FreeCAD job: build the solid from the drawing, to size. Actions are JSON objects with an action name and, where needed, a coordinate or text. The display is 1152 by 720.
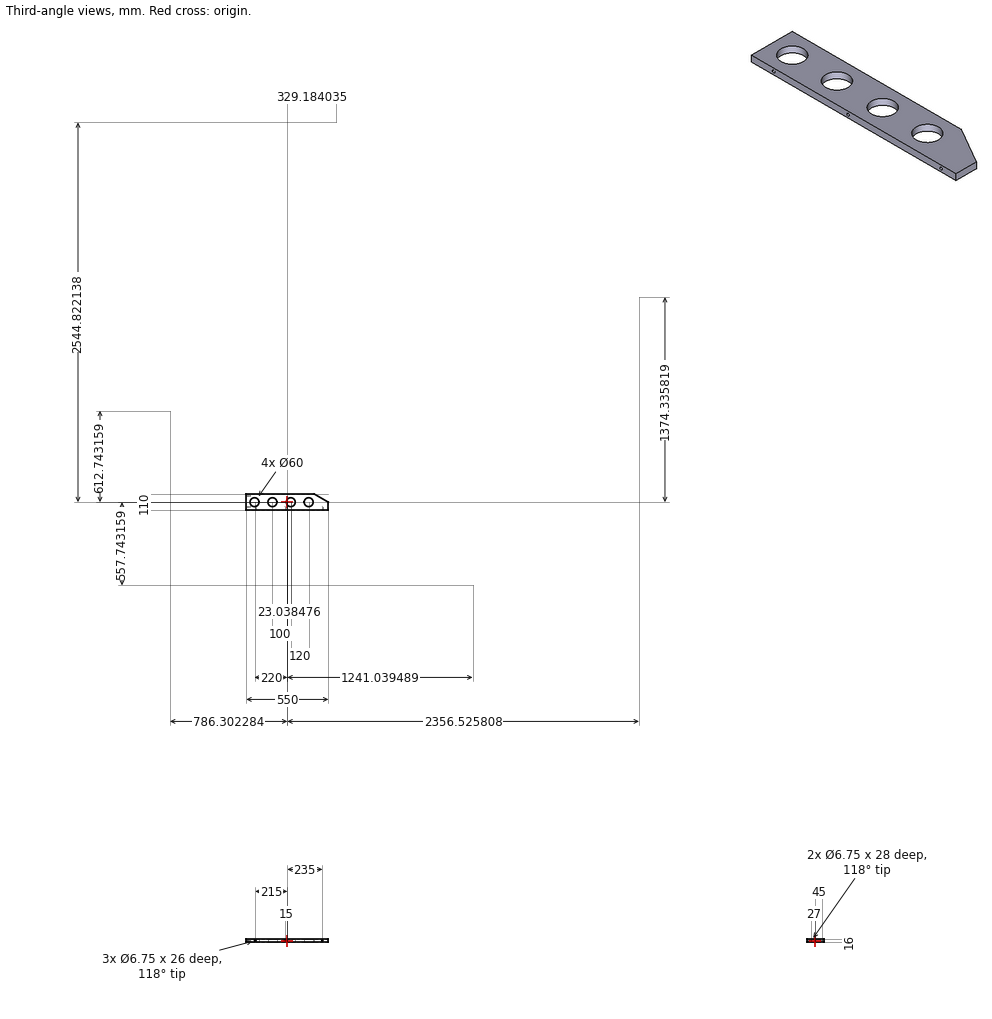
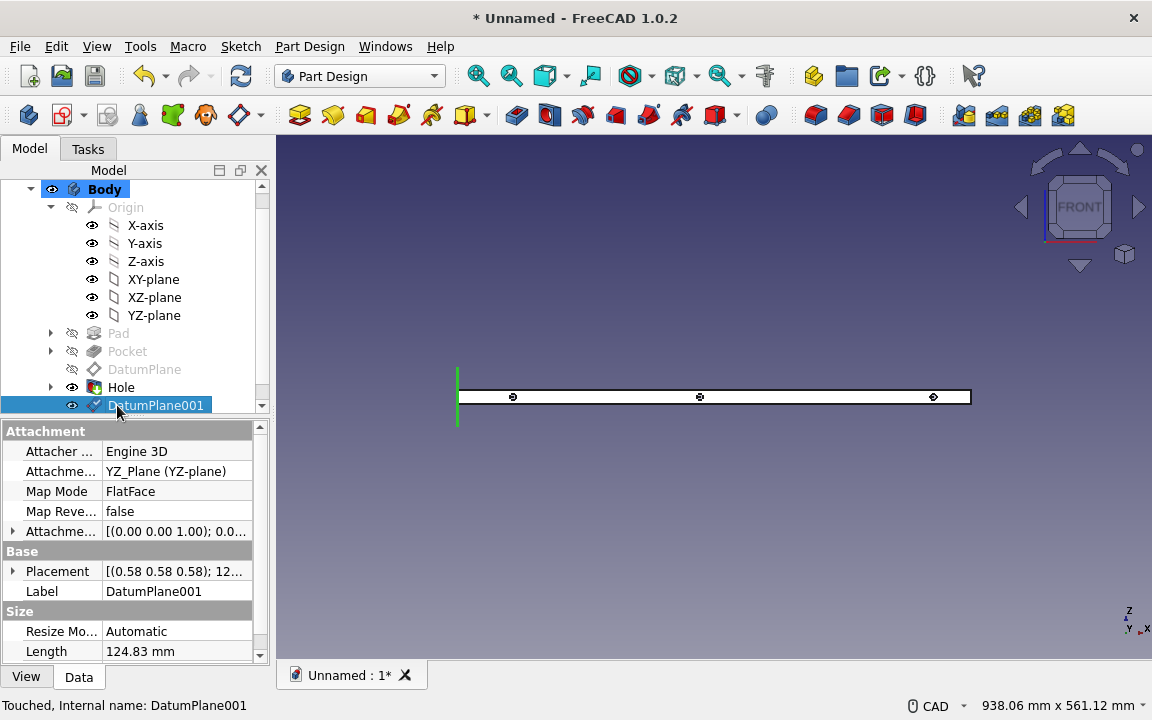
{"action": "left_click", "coordinate": [62, 116]}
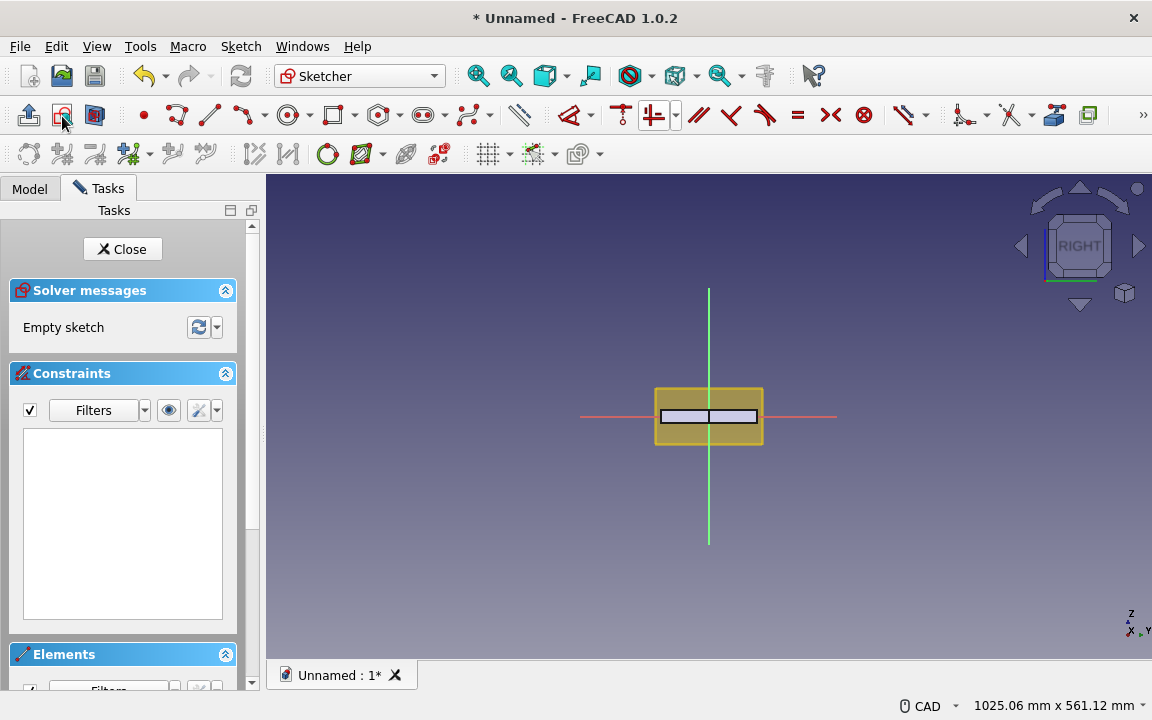
{"action": "key", "text": "q s"}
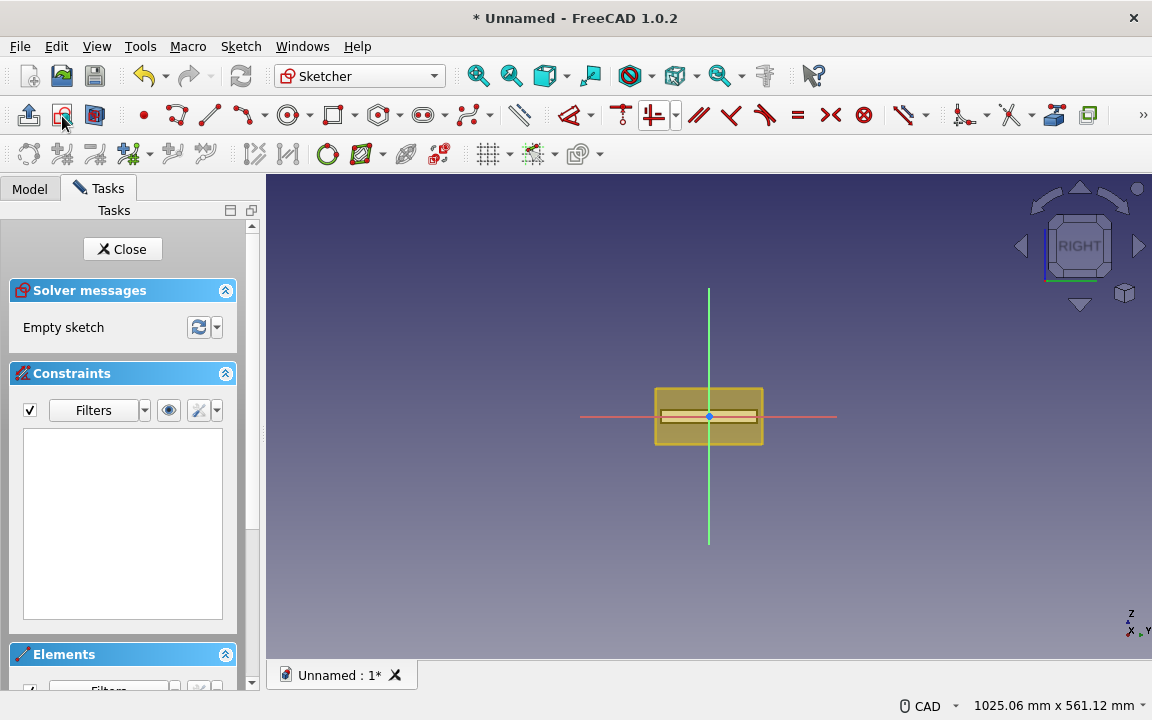
{"action": "scroll", "coordinate": [729, 416], "scroll_direction": "up", "scroll_amount": 10}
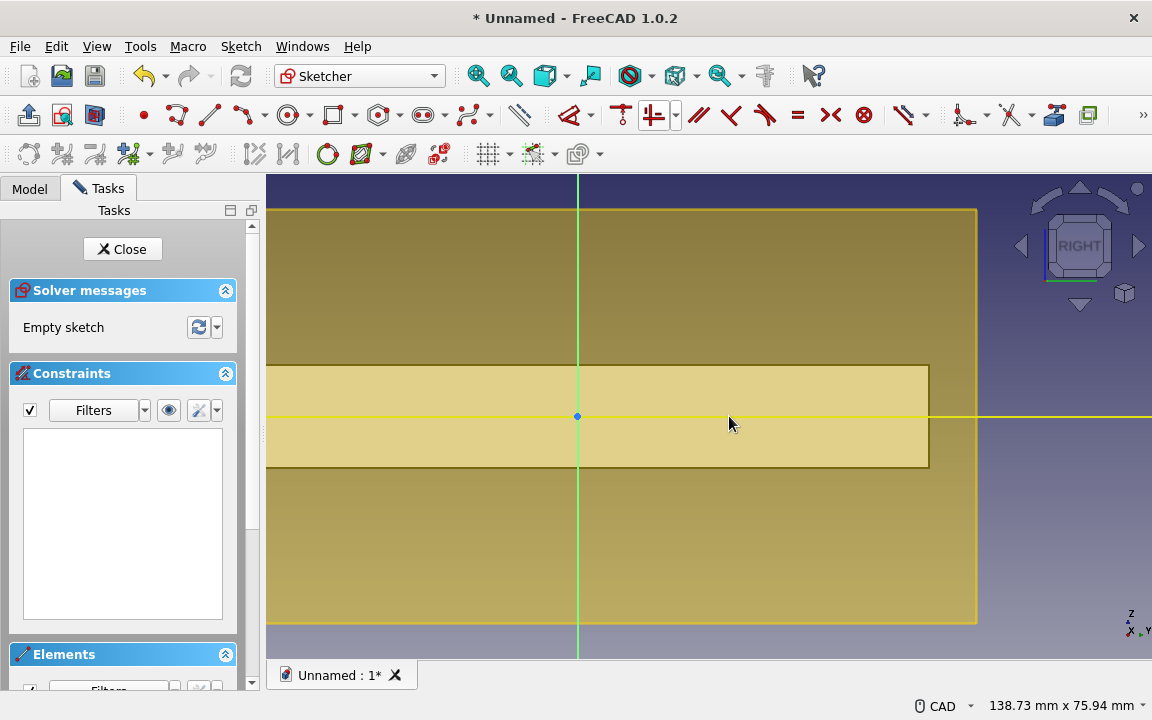
{"action": "key", "text": "g c"}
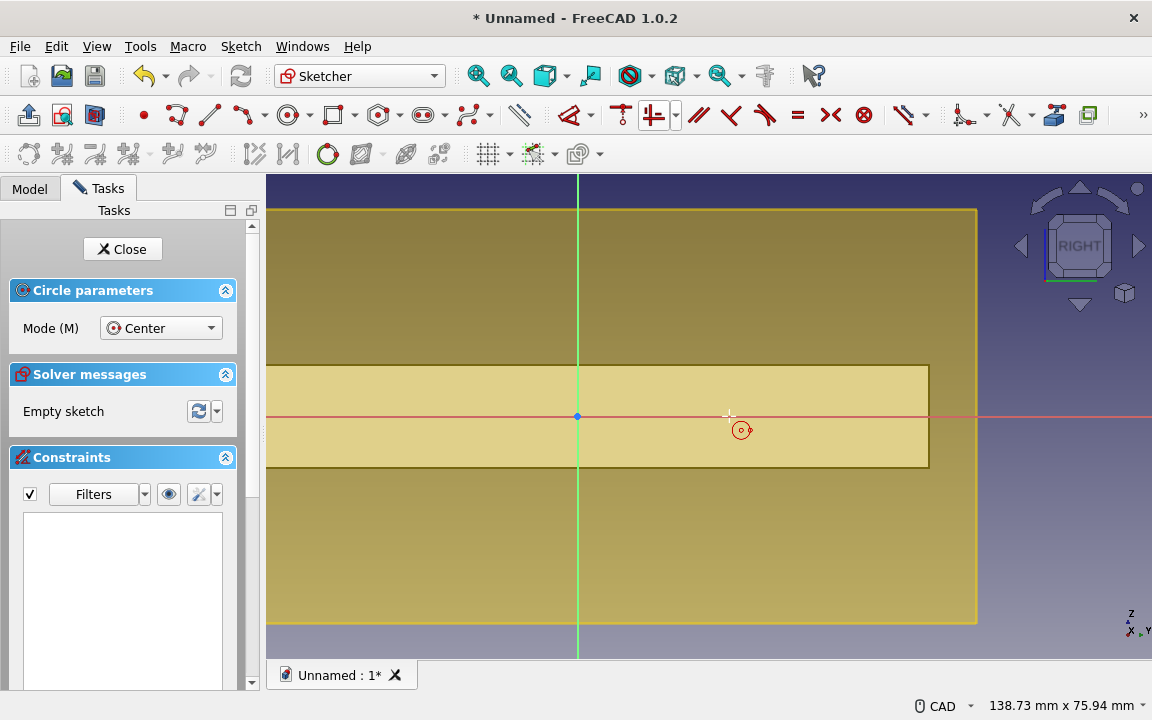
{"action": "left_click", "coordinate": [405, 416]}
{"action": "mouse_move", "coordinate": [421, 401]}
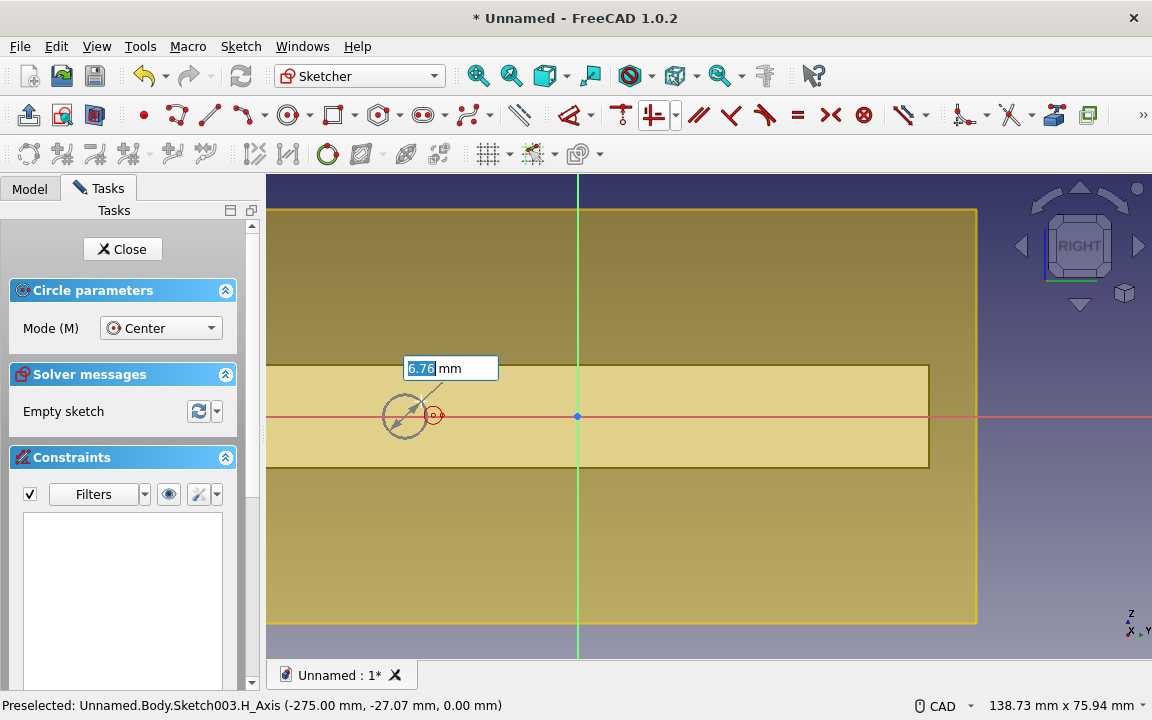
{"action": "type", "text": "6.75"}
{"action": "key", "text": "Return"}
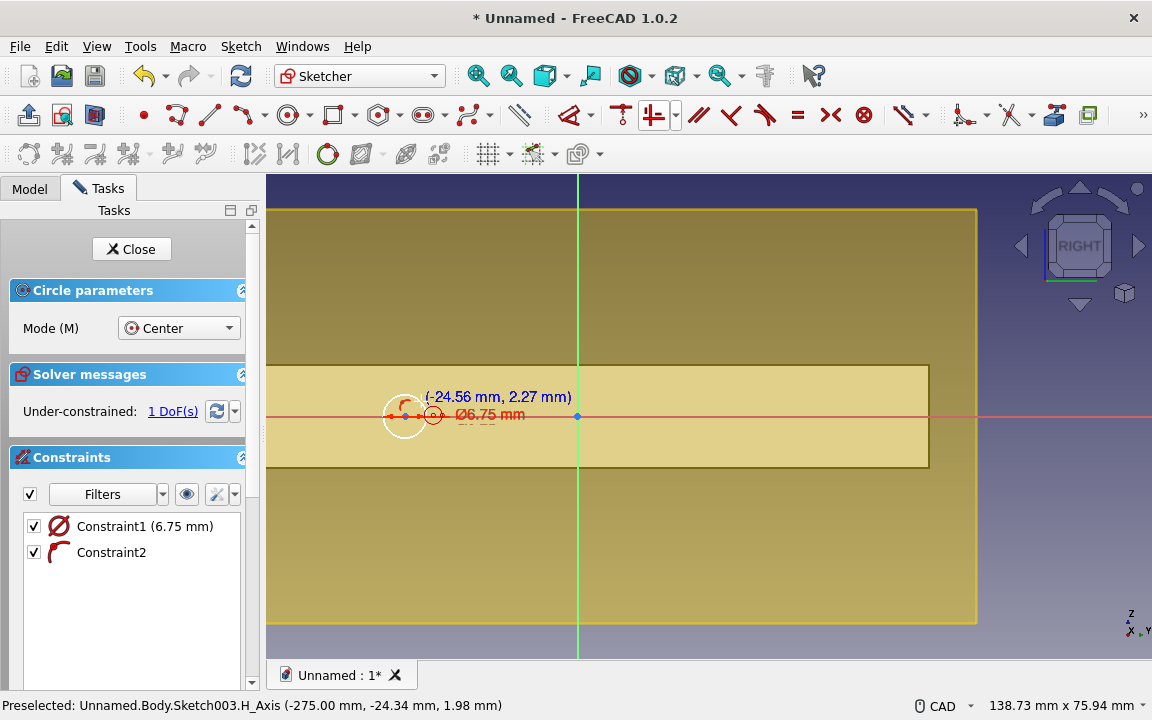
{"action": "left_click", "coordinate": [865, 416]}
{"action": "mouse_move", "coordinate": [881, 401]}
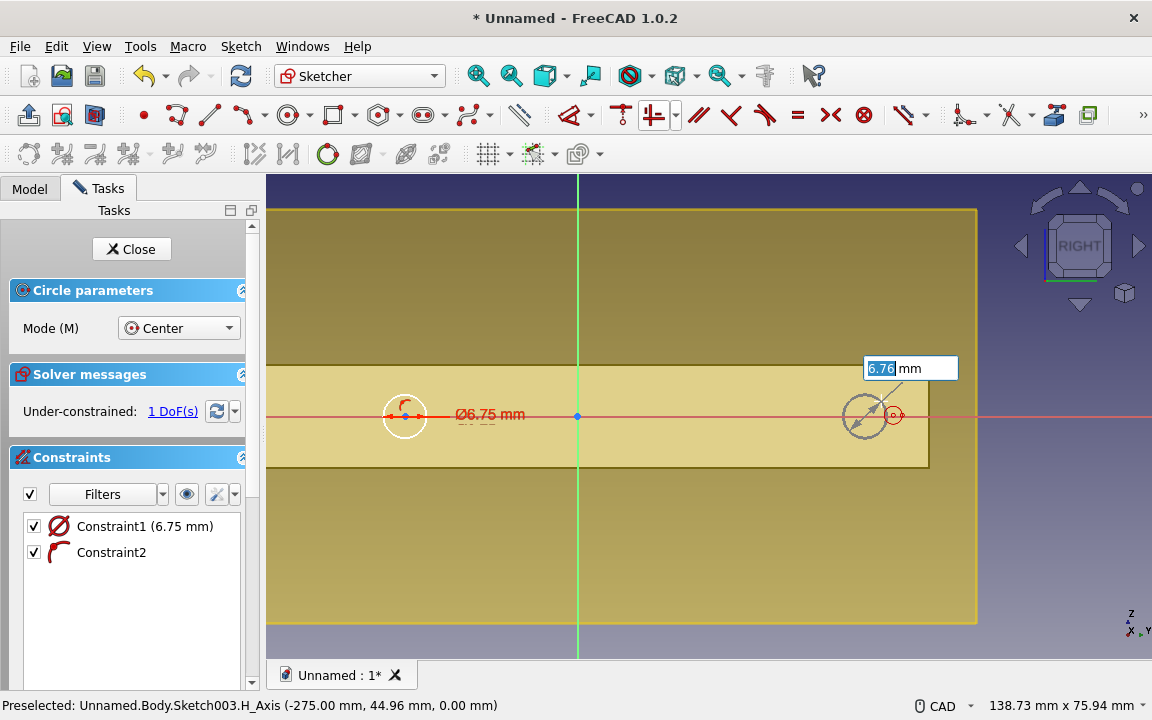
{"action": "type", "text": "6.75"}
{"action": "key", "text": "Return"}
{"action": "key", "text": "Escape"}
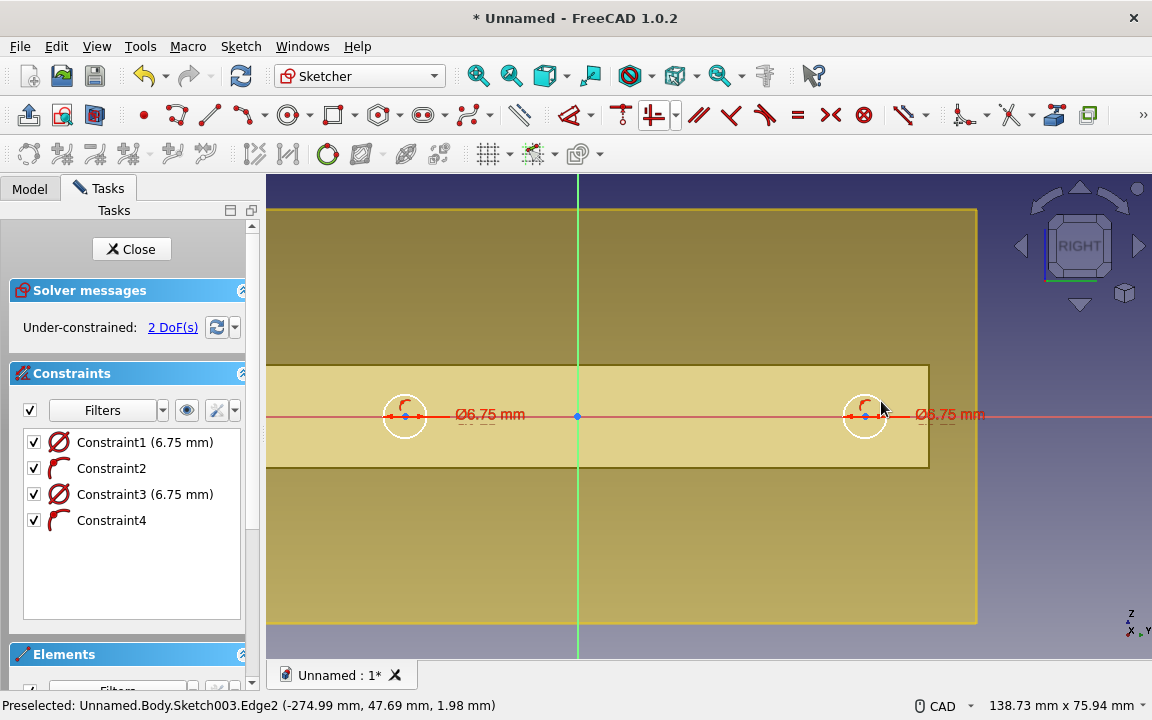
{"action": "key", "text": "d"}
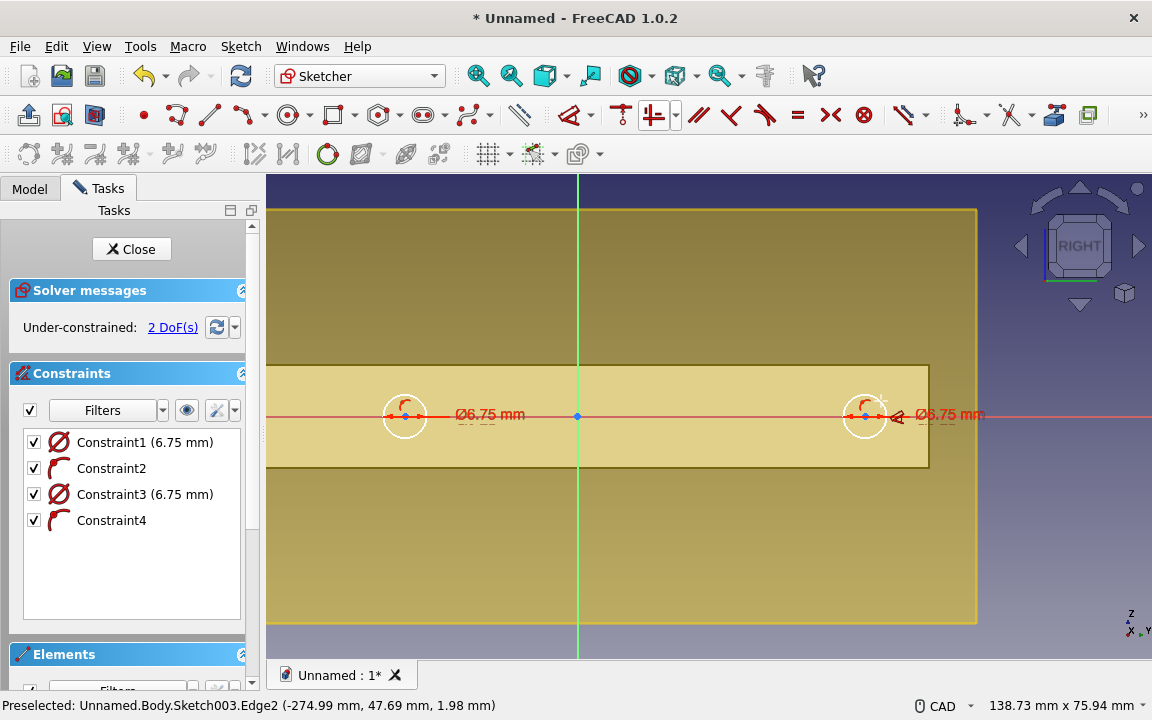
{"action": "left_click", "coordinate": [405, 416]}
{"action": "left_click", "coordinate": [491, 450]}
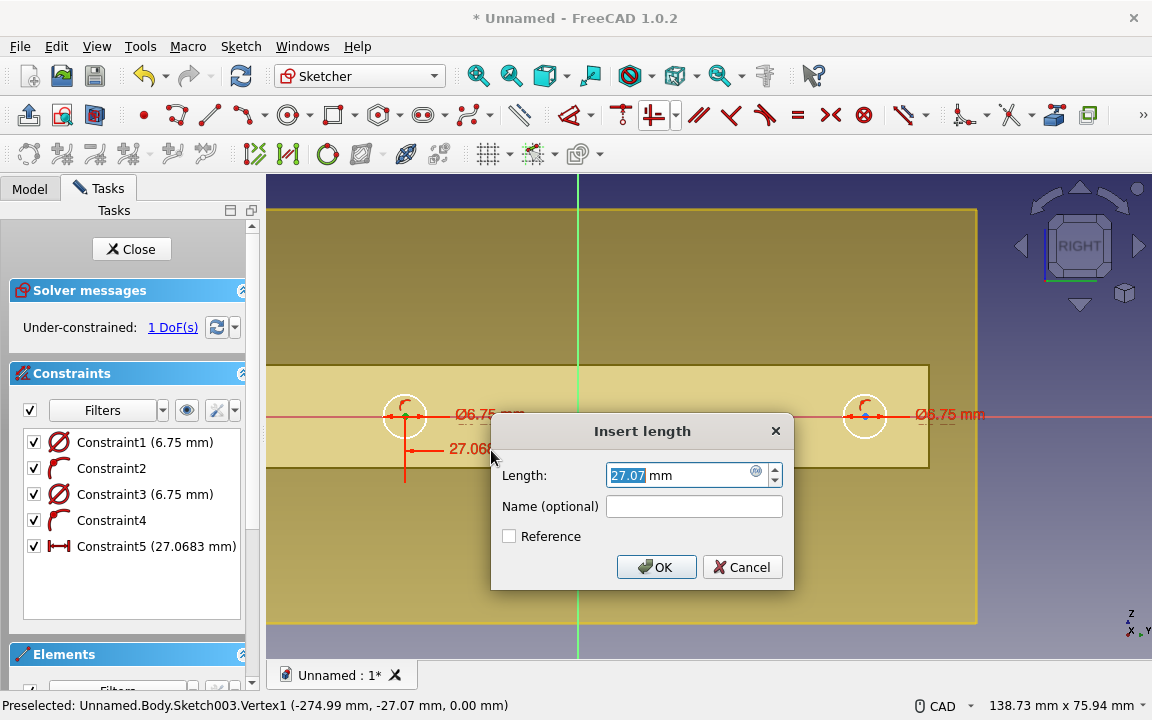
{"action": "type", "text": "27"}
{"action": "key", "text": "Return"}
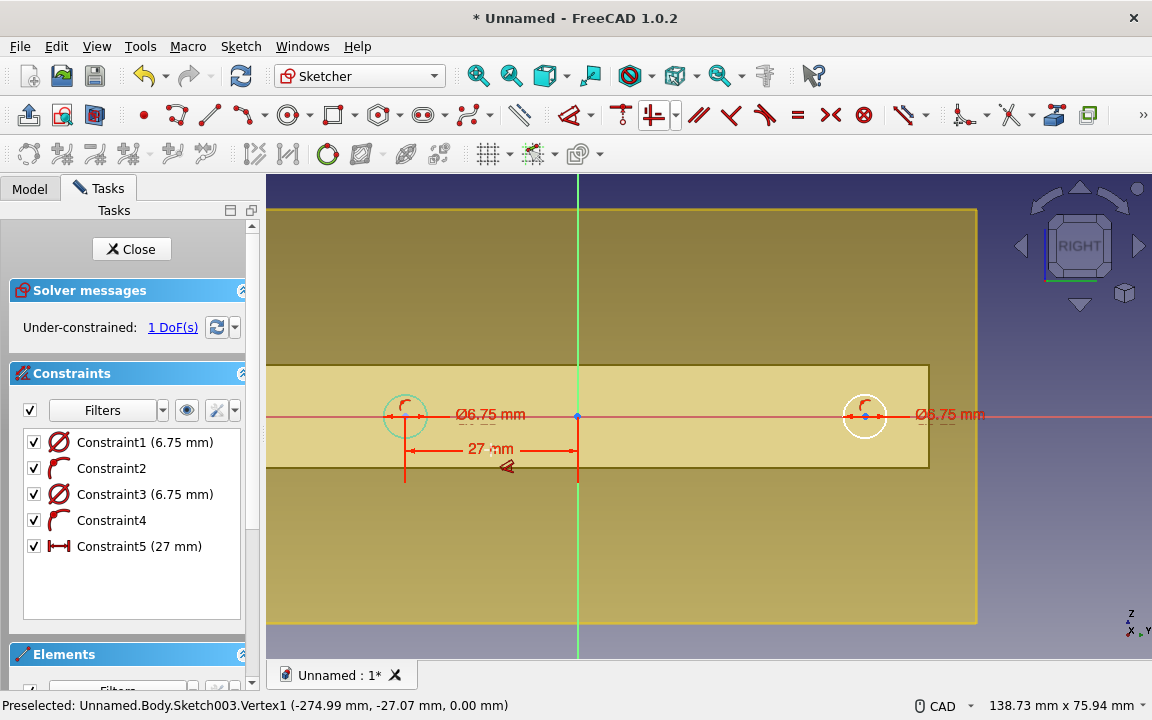
{"action": "left_click", "coordinate": [865, 416]}
{"action": "left_click", "coordinate": [721, 450]}